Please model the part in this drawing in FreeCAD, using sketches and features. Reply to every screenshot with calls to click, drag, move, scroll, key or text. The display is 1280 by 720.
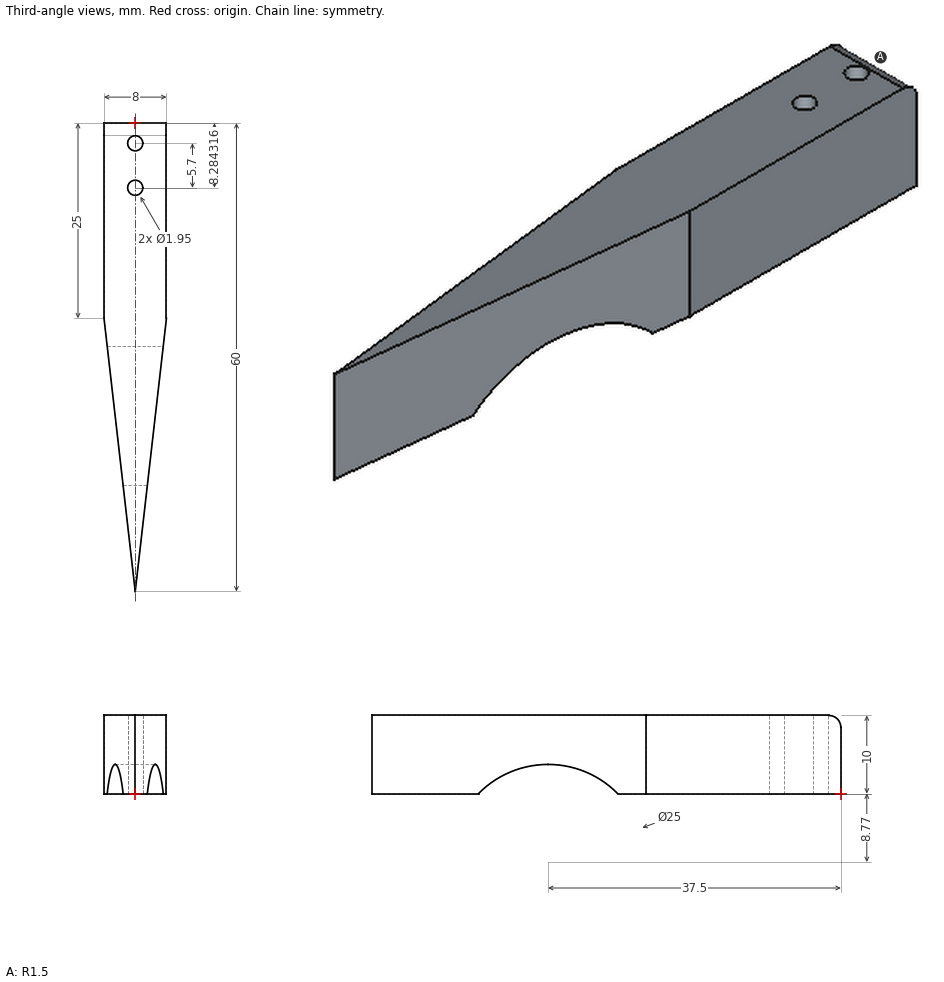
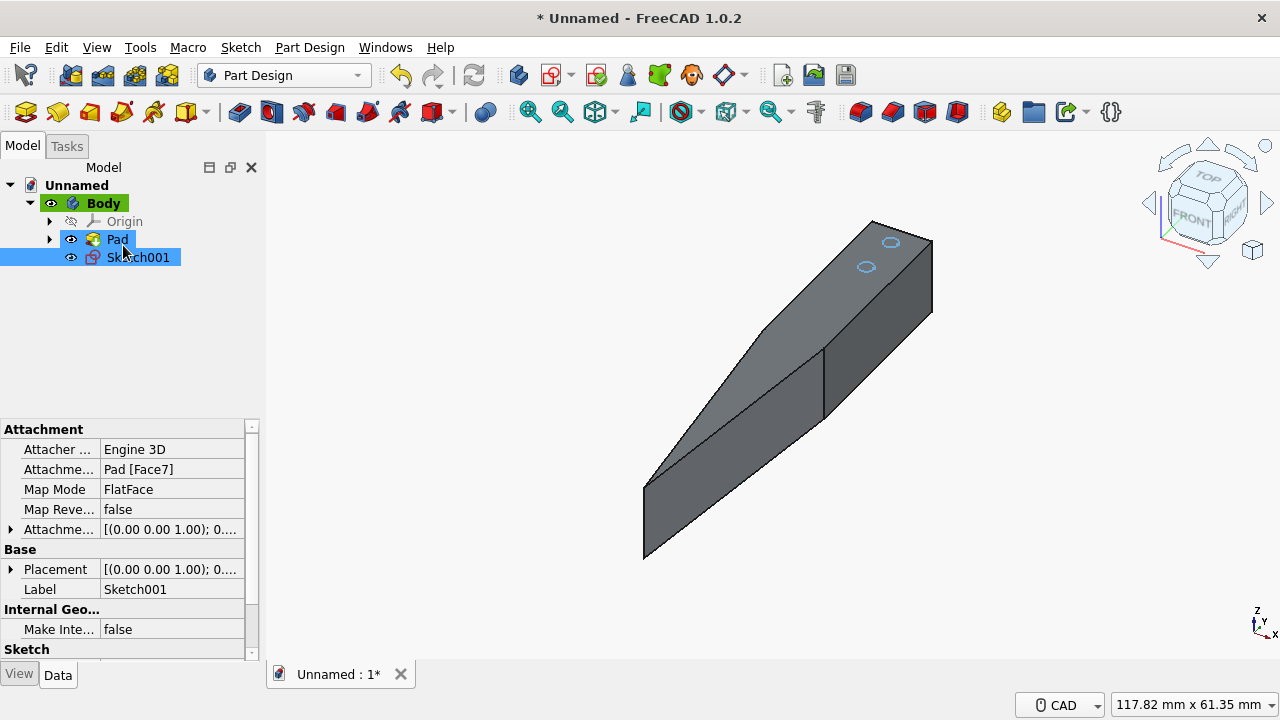
click(240, 112)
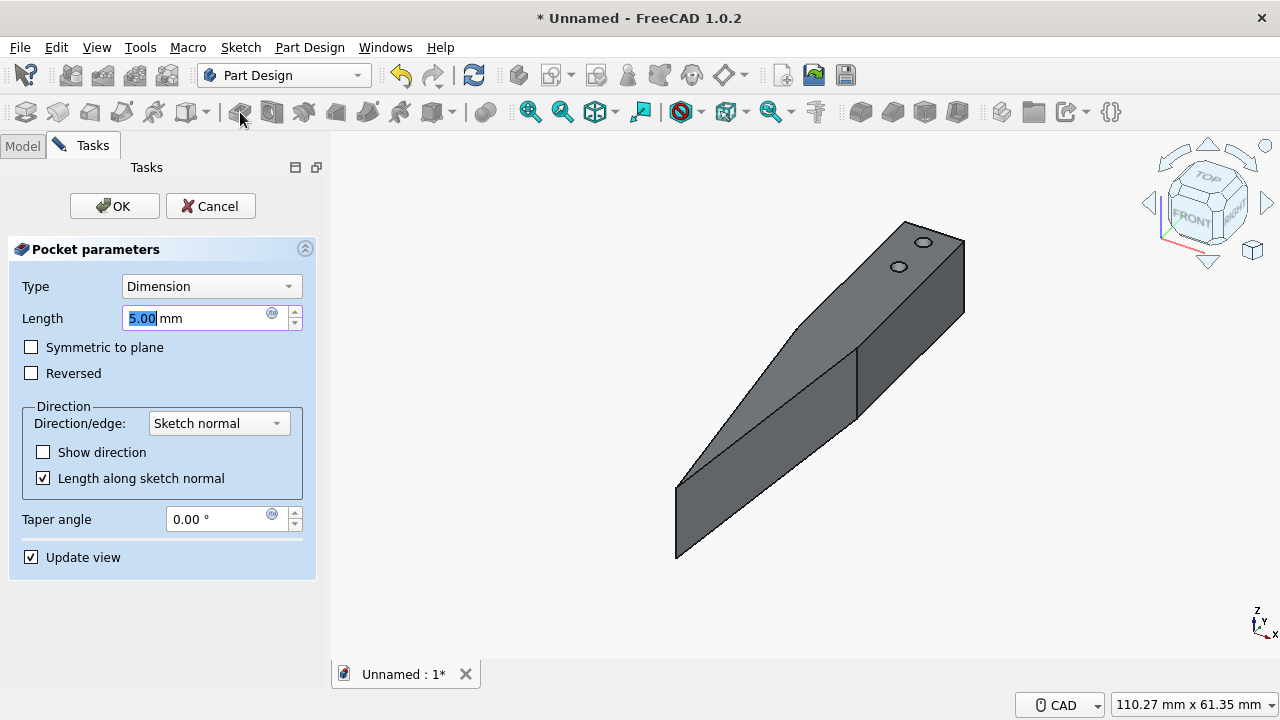
click(212, 286)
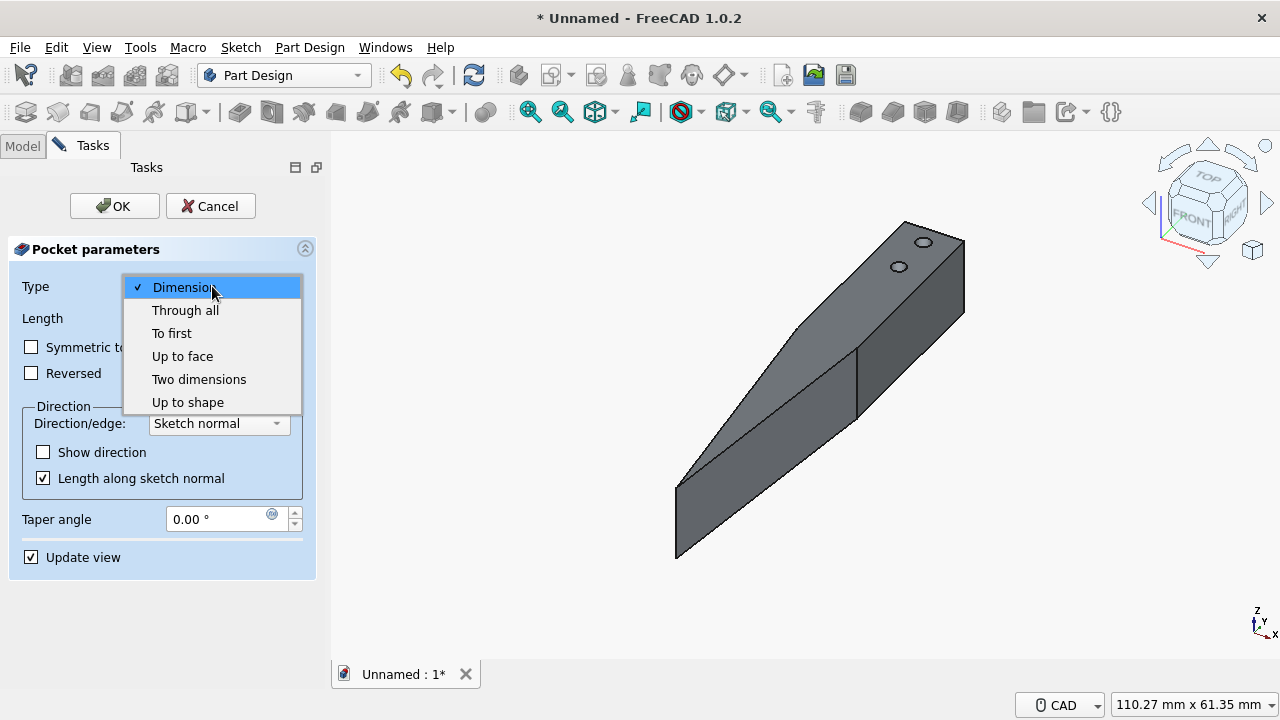
click(212, 310)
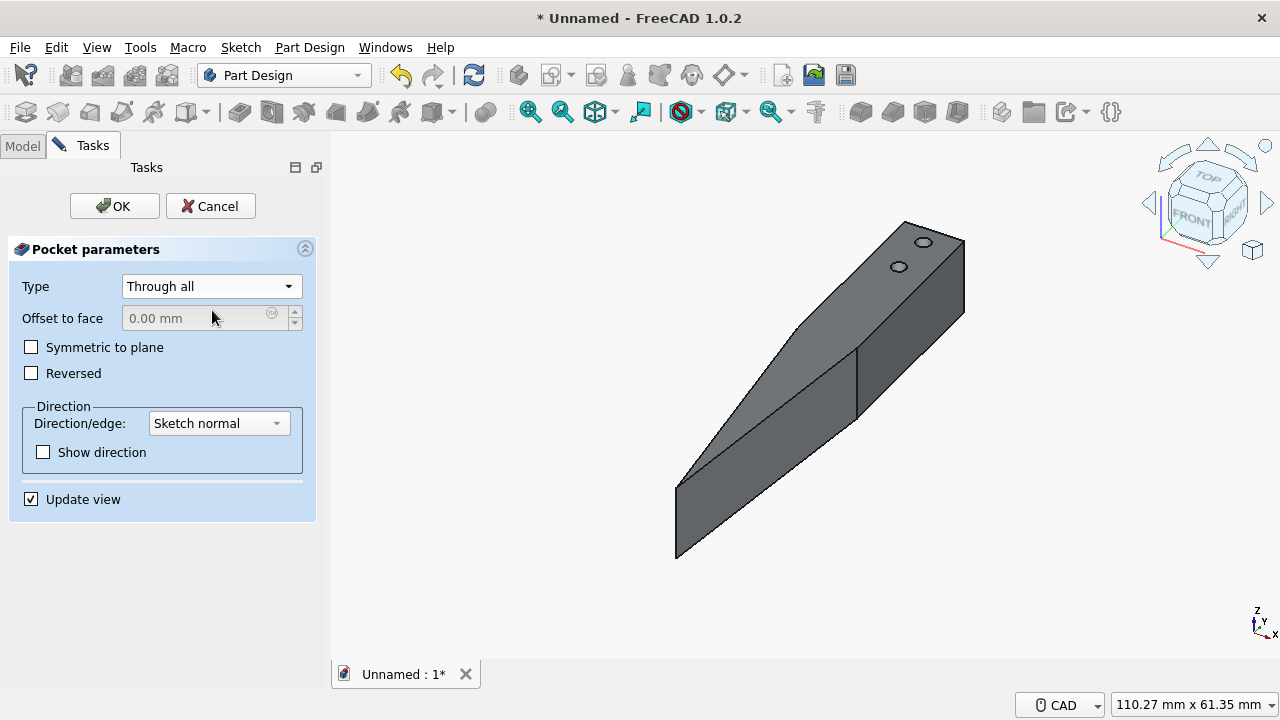
click(115, 206)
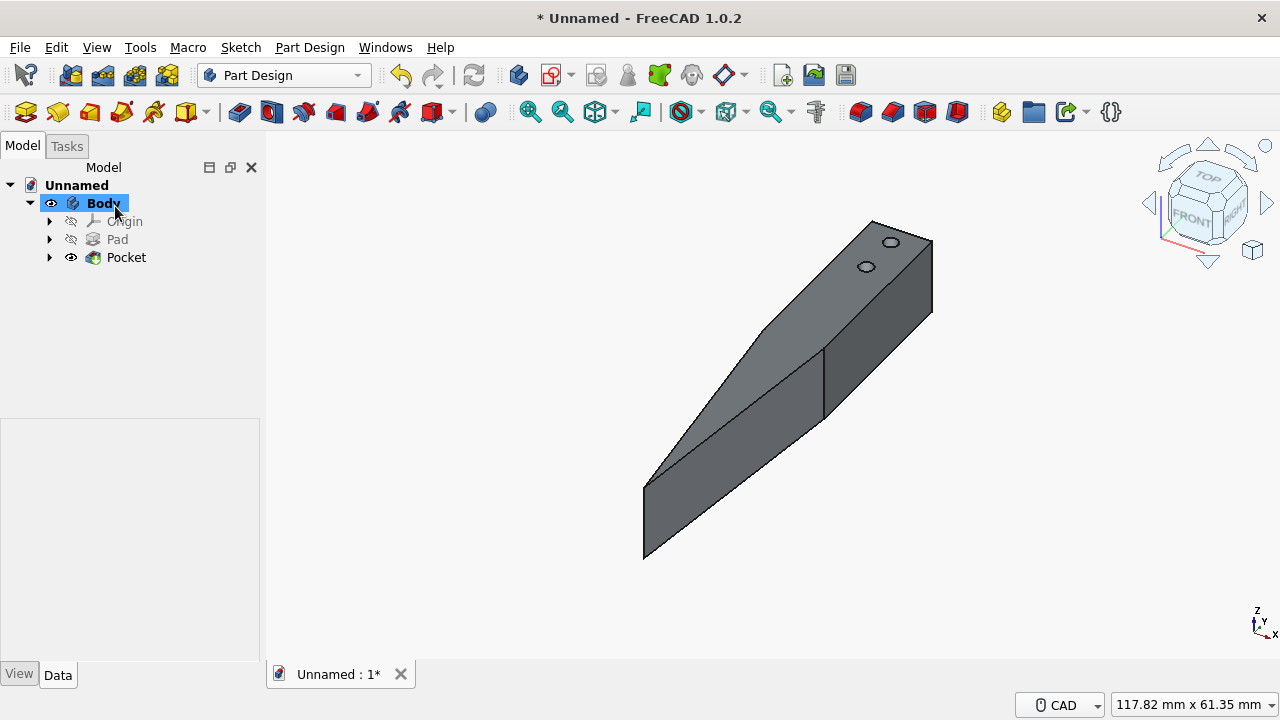
key(0)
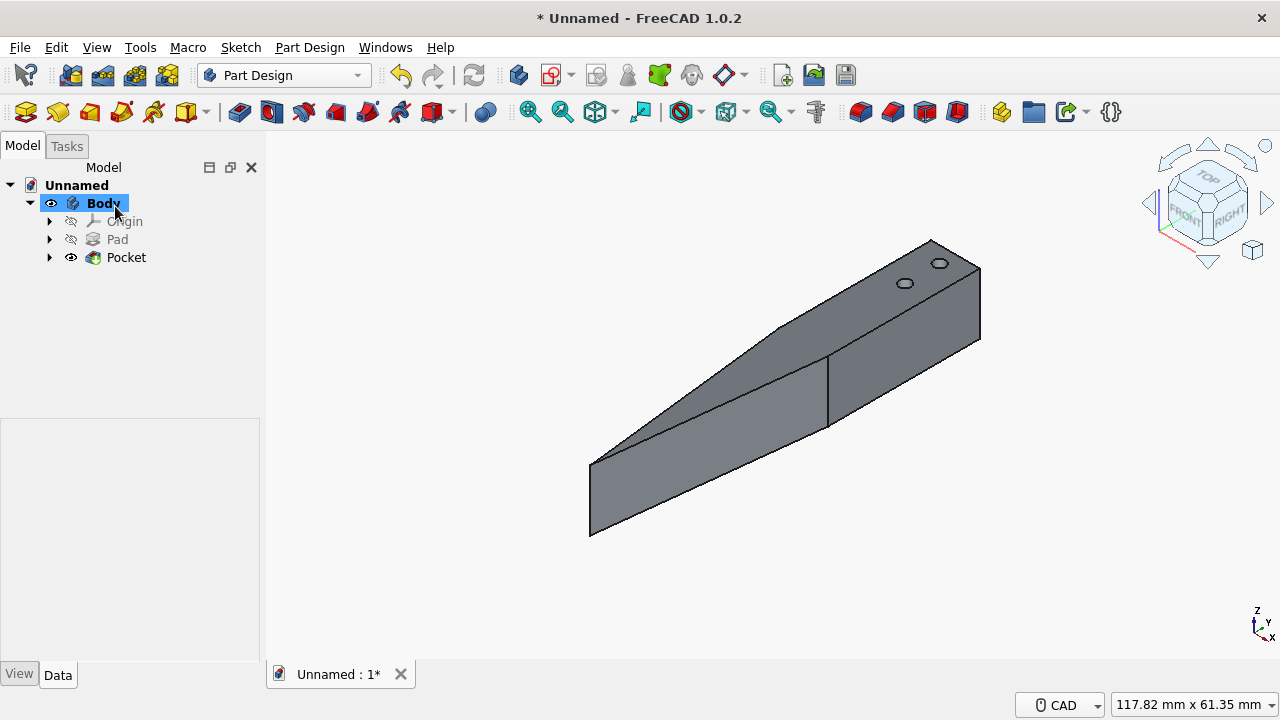
key(2)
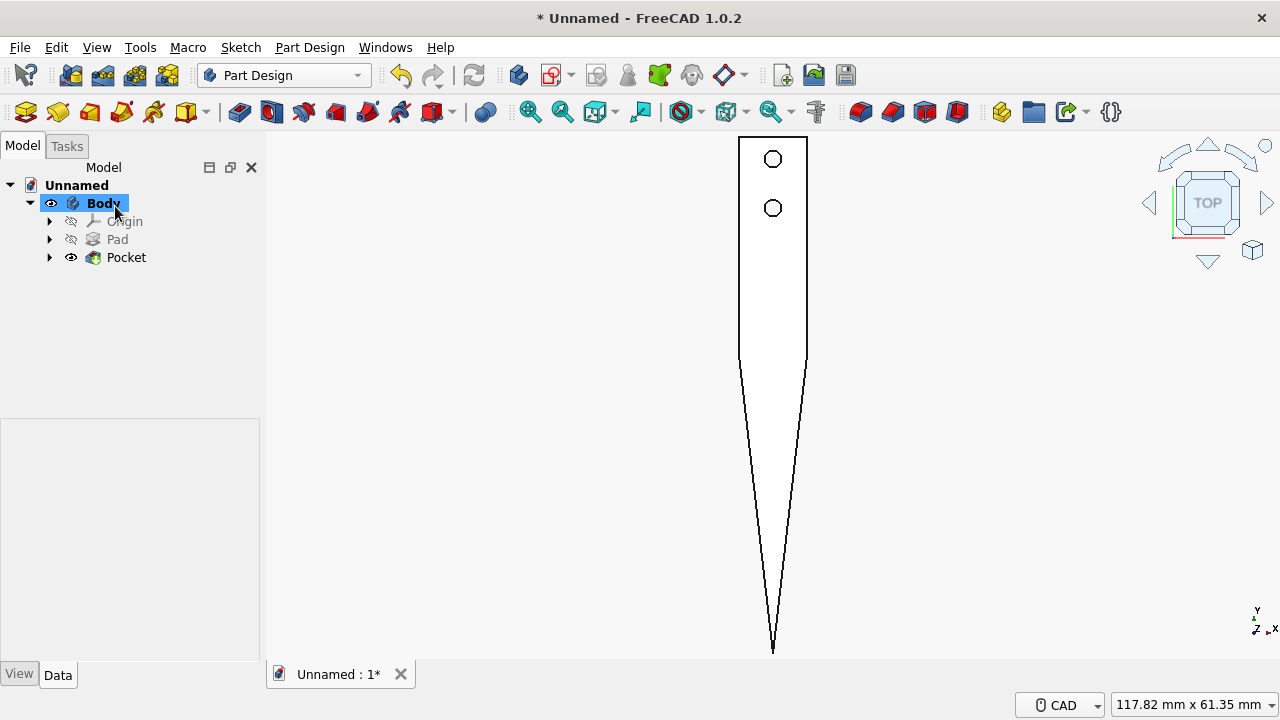
key(1)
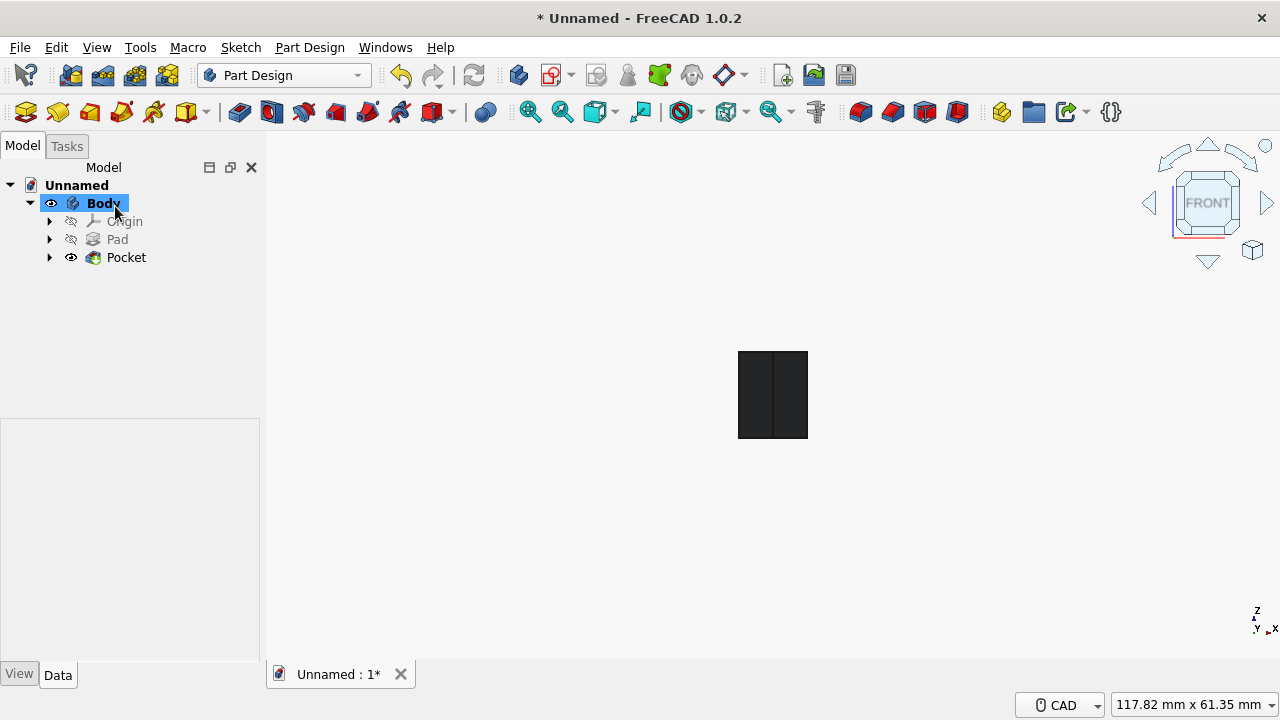
key(v)
key(f)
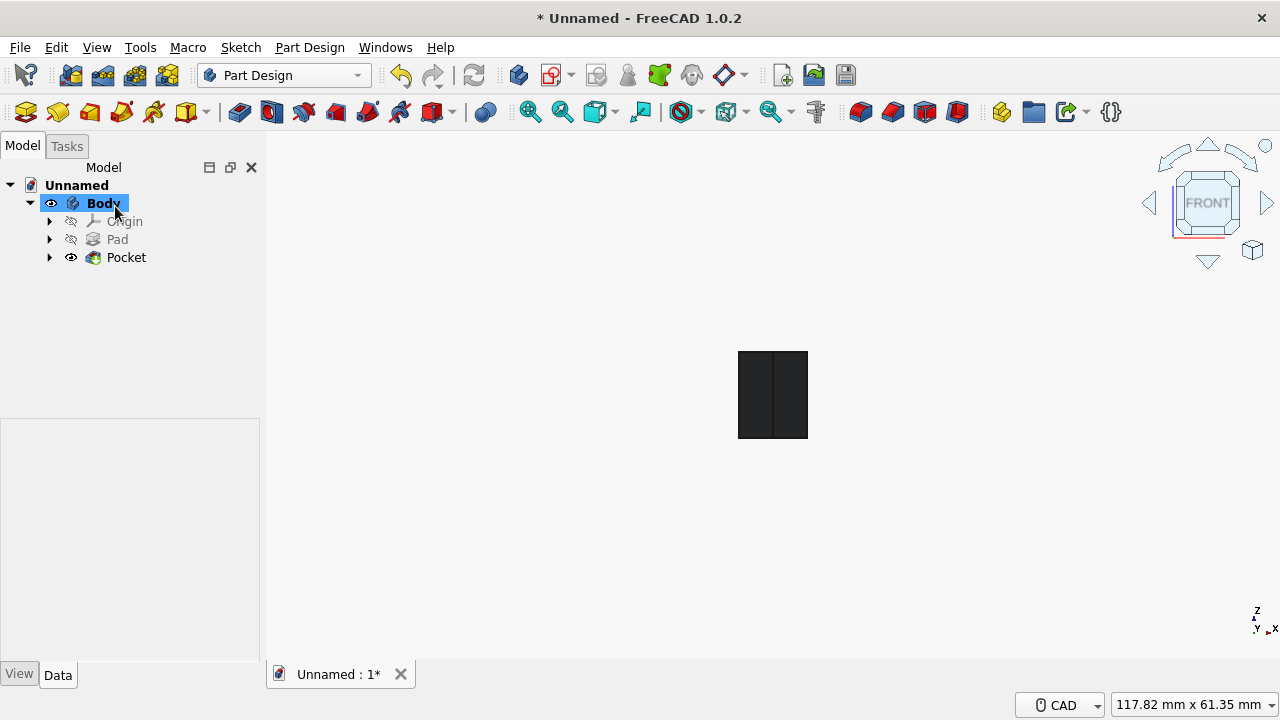
key(3)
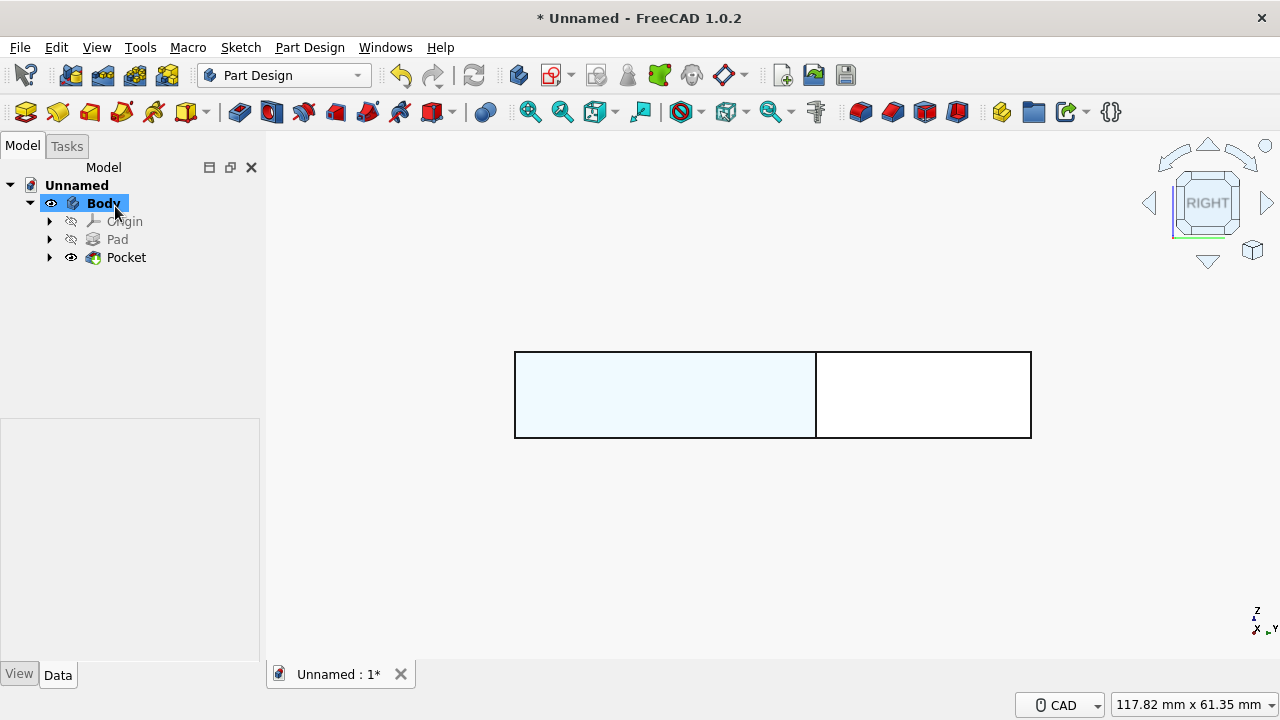
key(5)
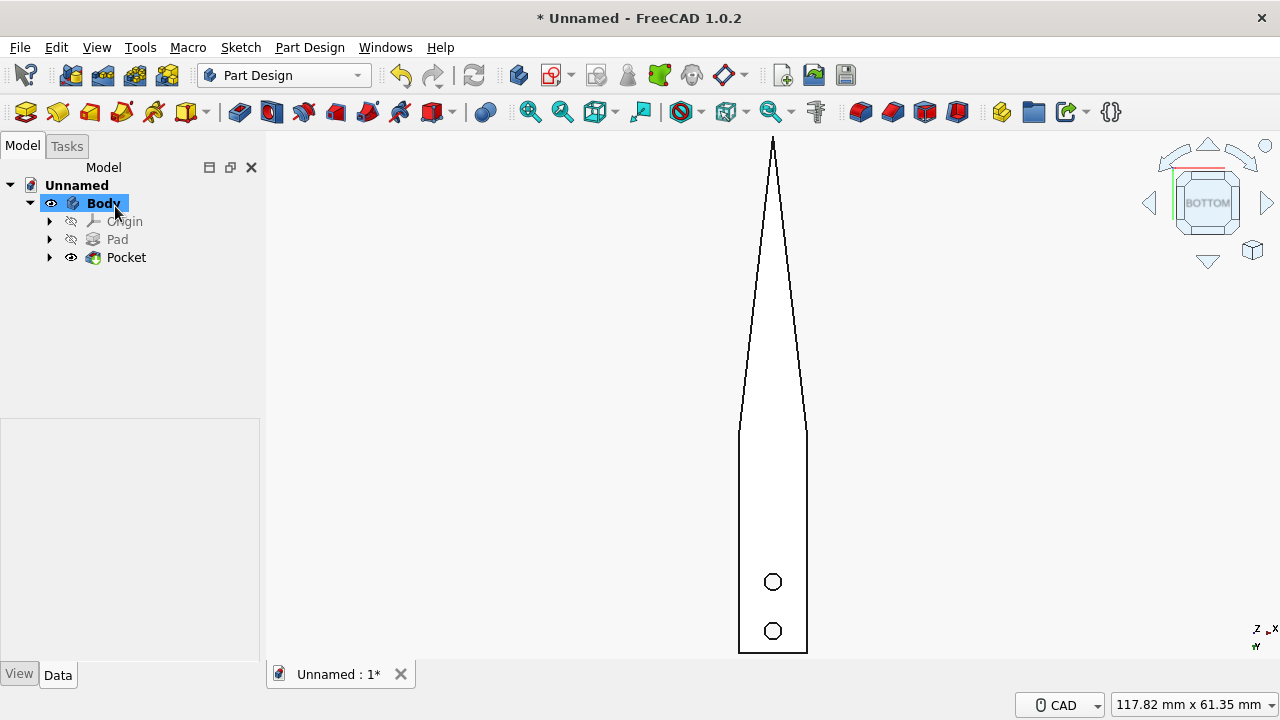
key(4)